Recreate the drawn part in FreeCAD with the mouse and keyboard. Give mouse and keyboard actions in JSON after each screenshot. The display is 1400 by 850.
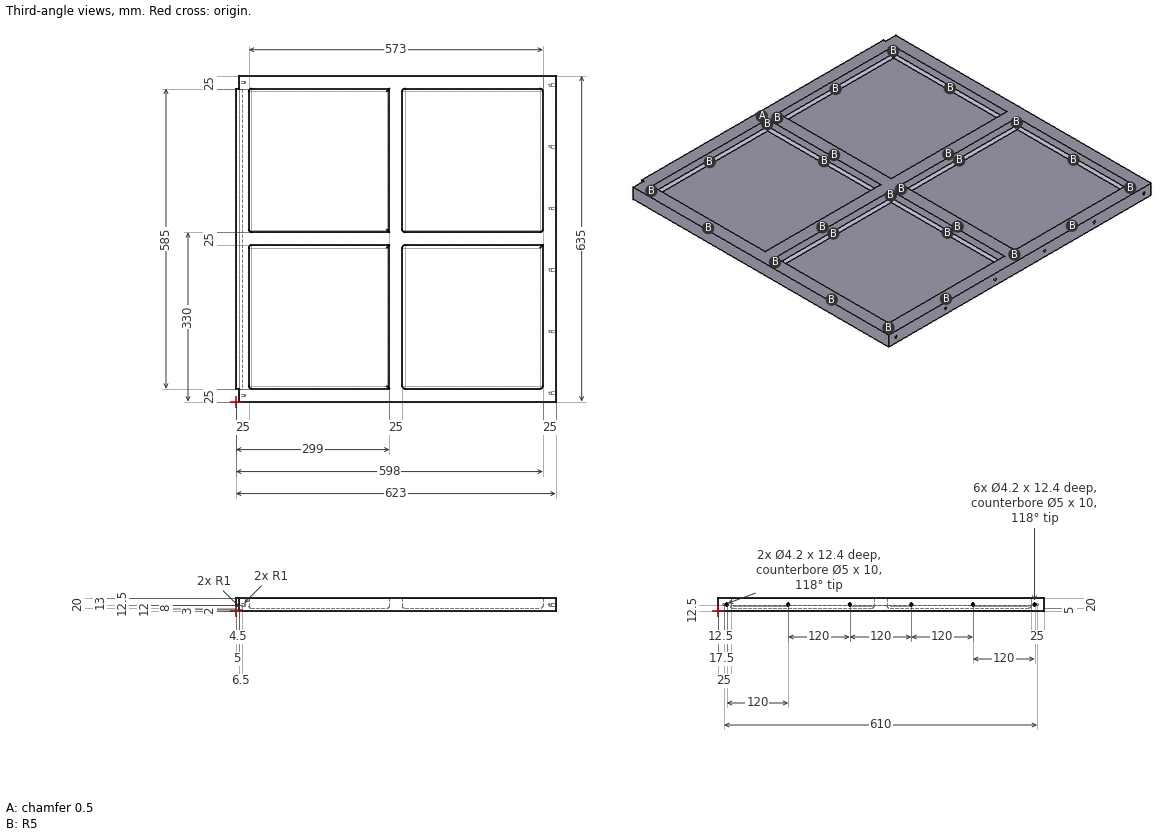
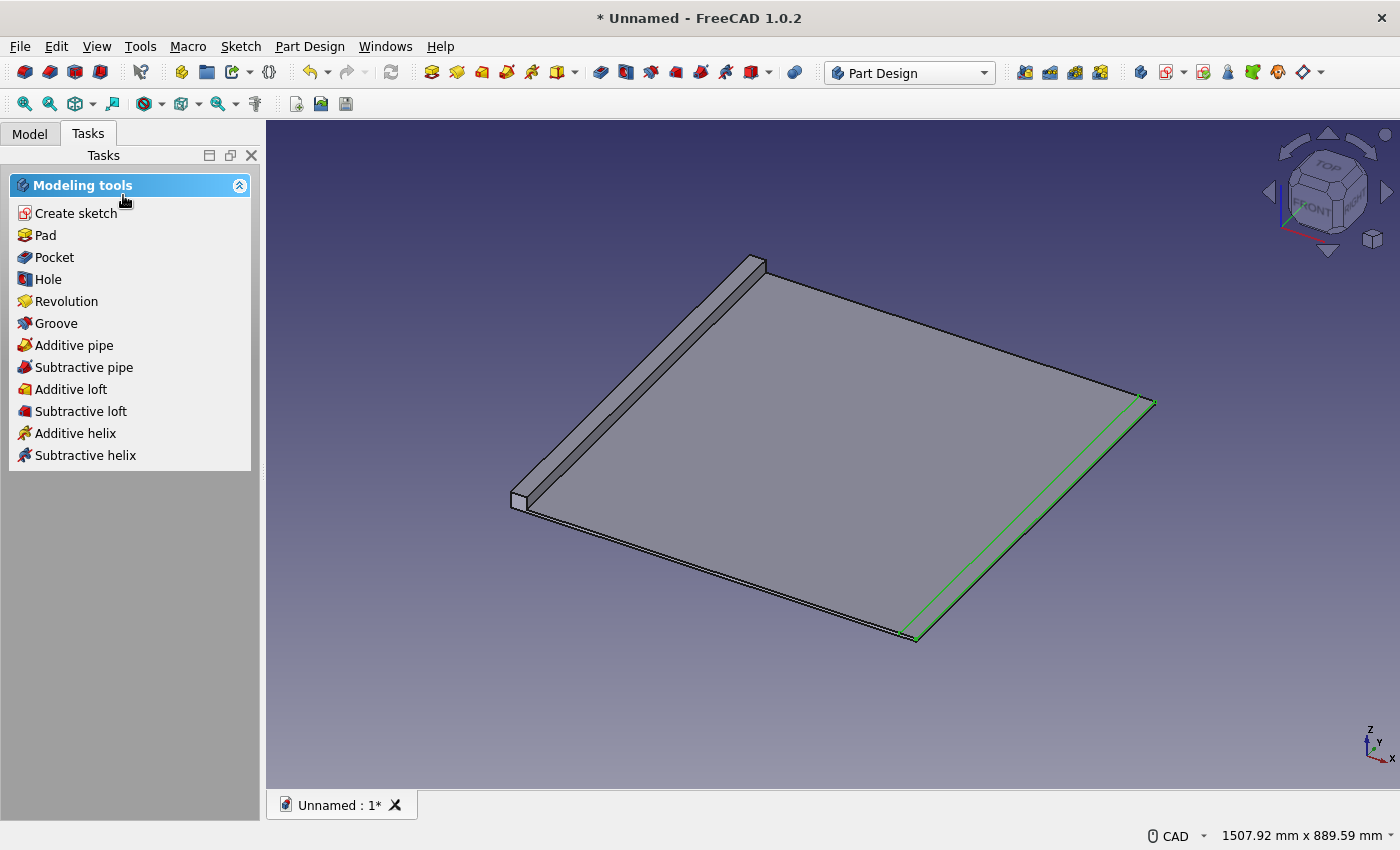
{"action": "left_click", "coordinate": [432, 72]}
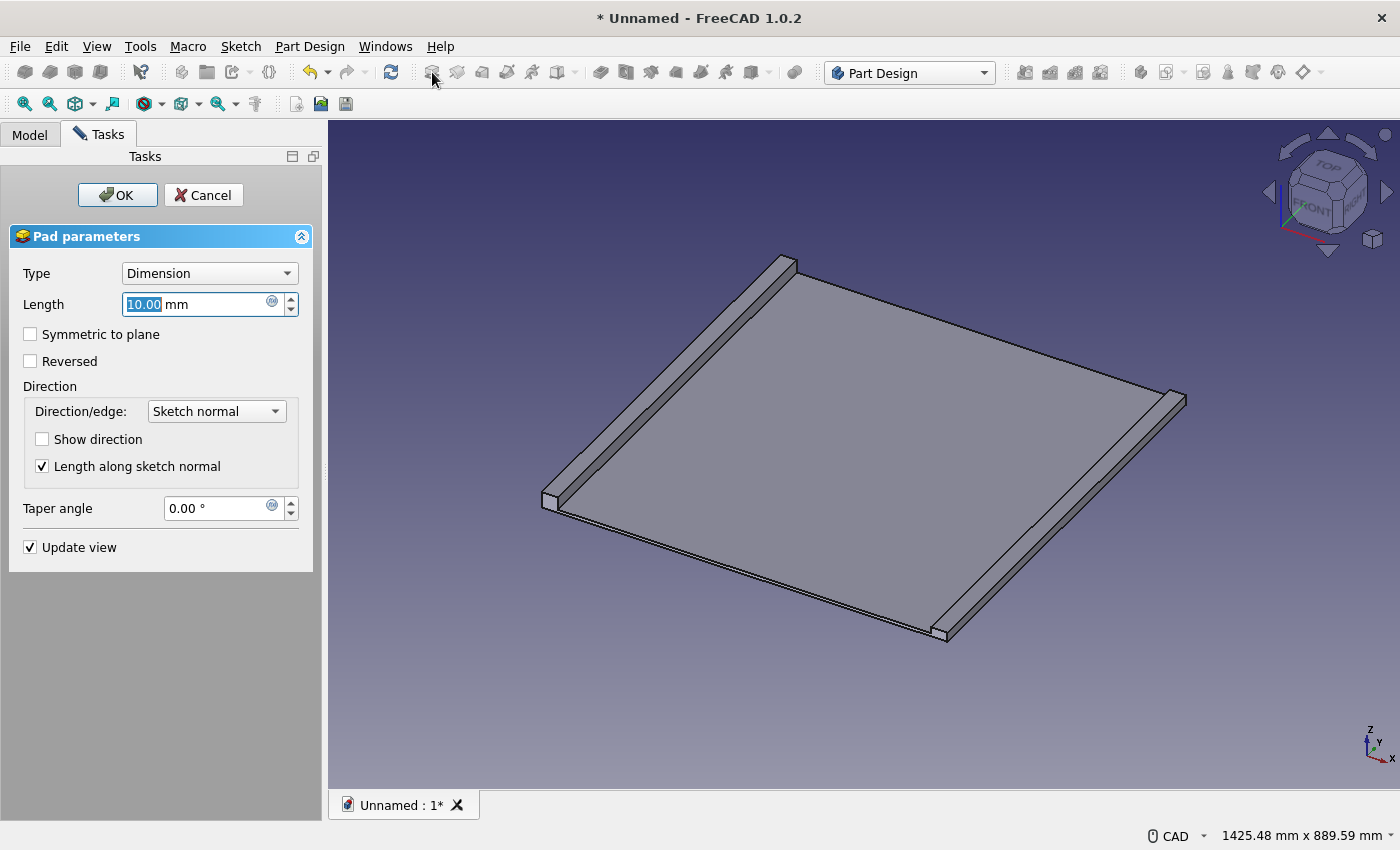
{"action": "type", "text": "20"}
{"action": "key", "text": "Tab"}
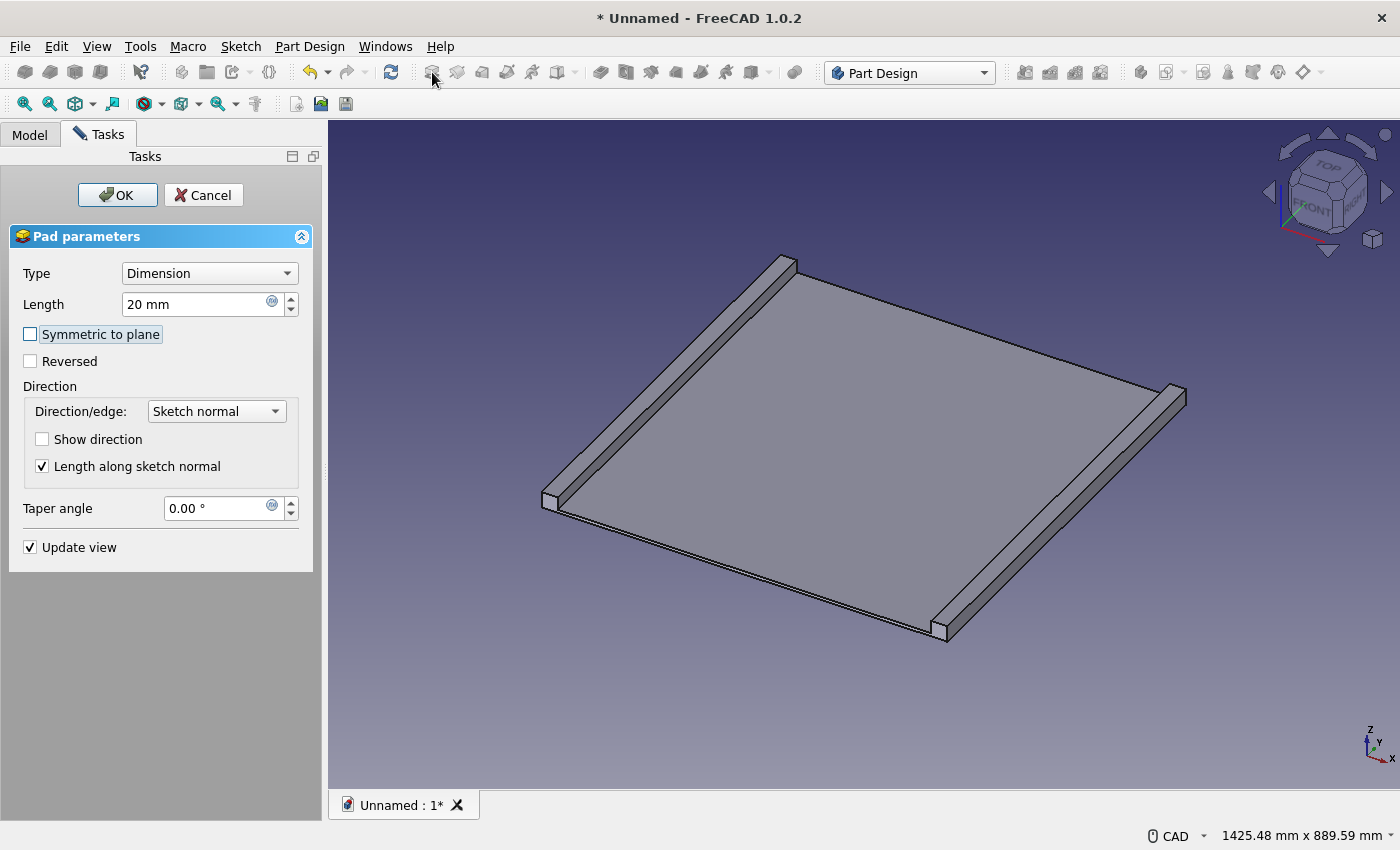
{"action": "left_click", "coordinate": [118, 195]}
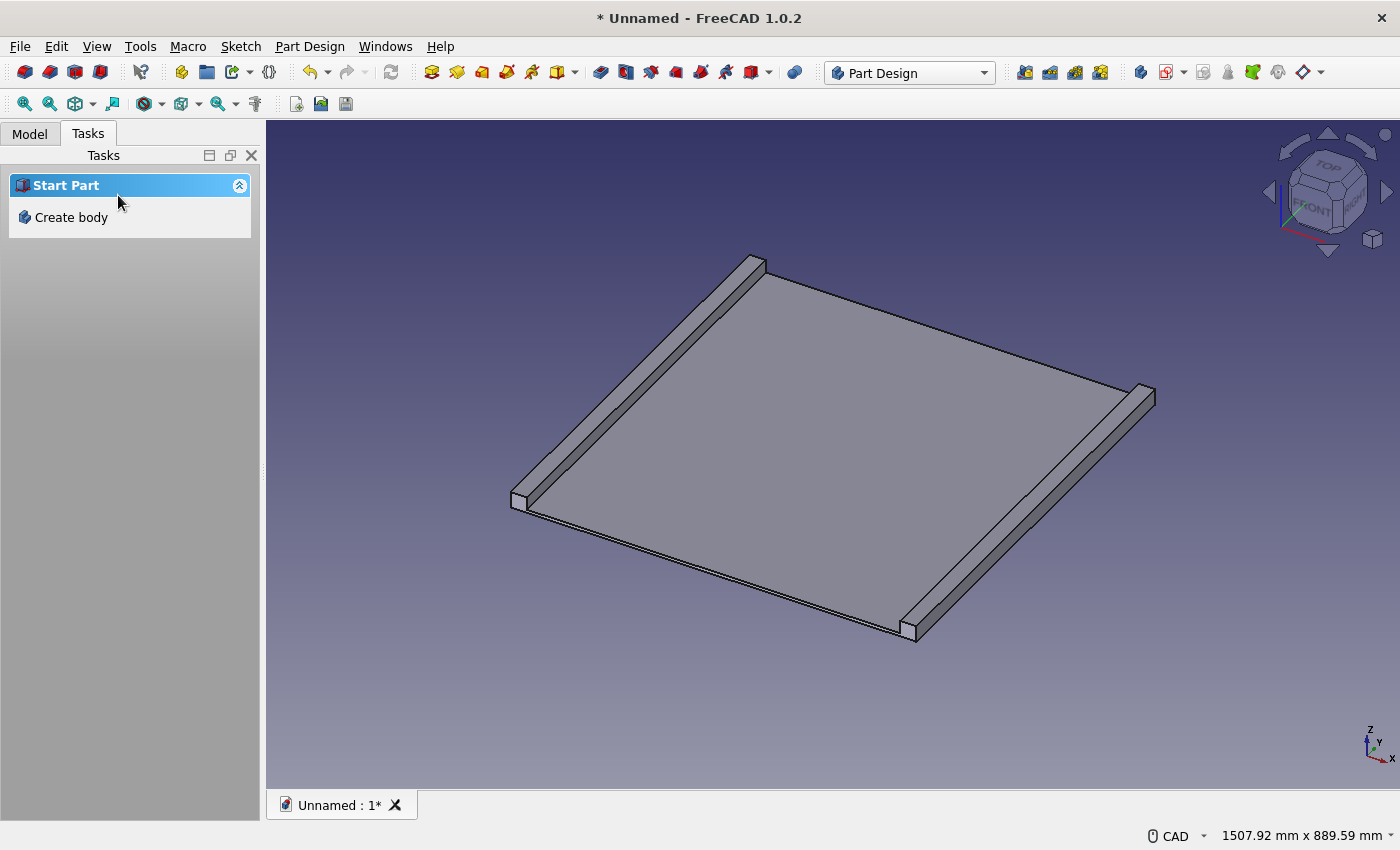
{"action": "key", "text": "4"}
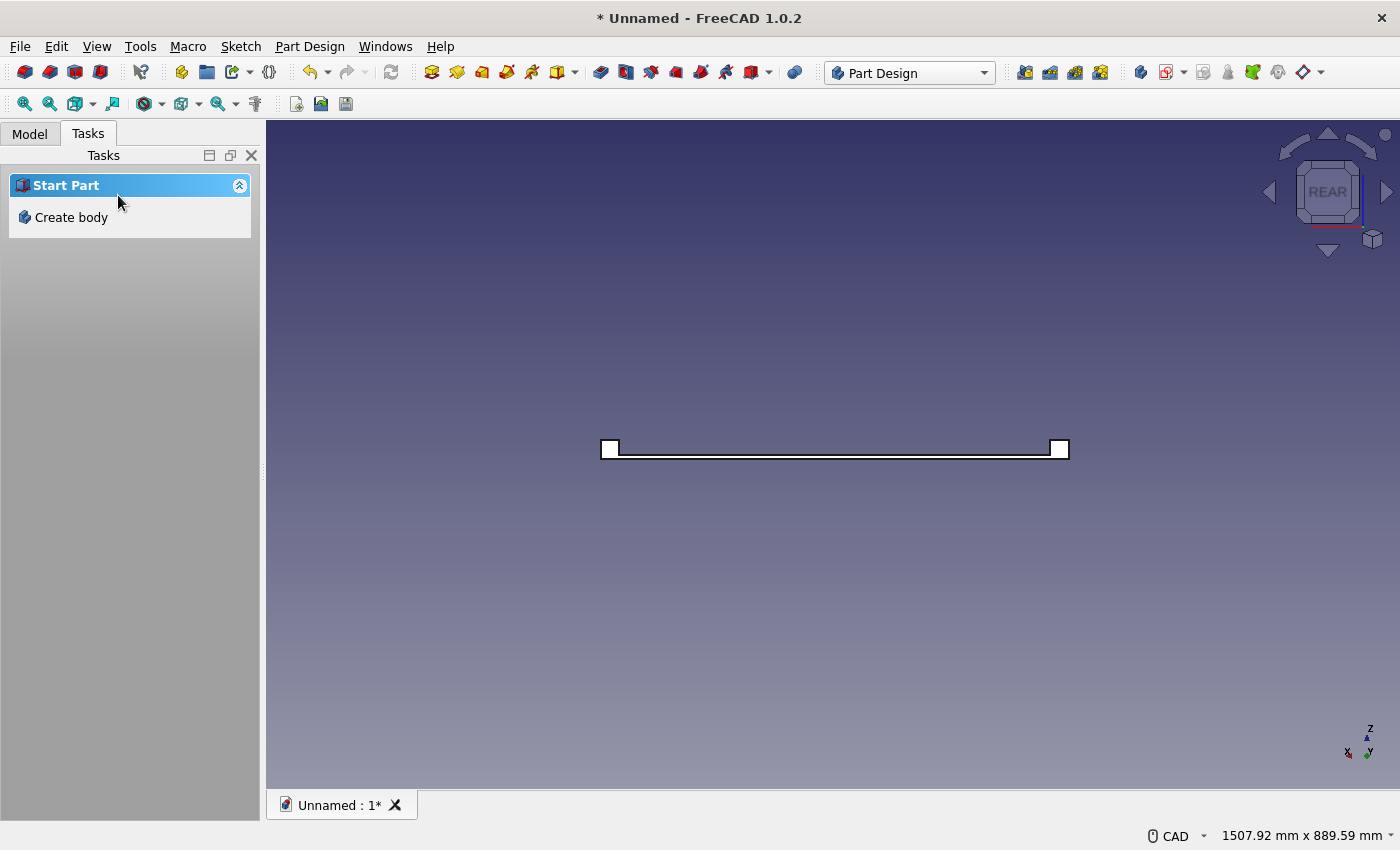
{"action": "key", "text": "v f"}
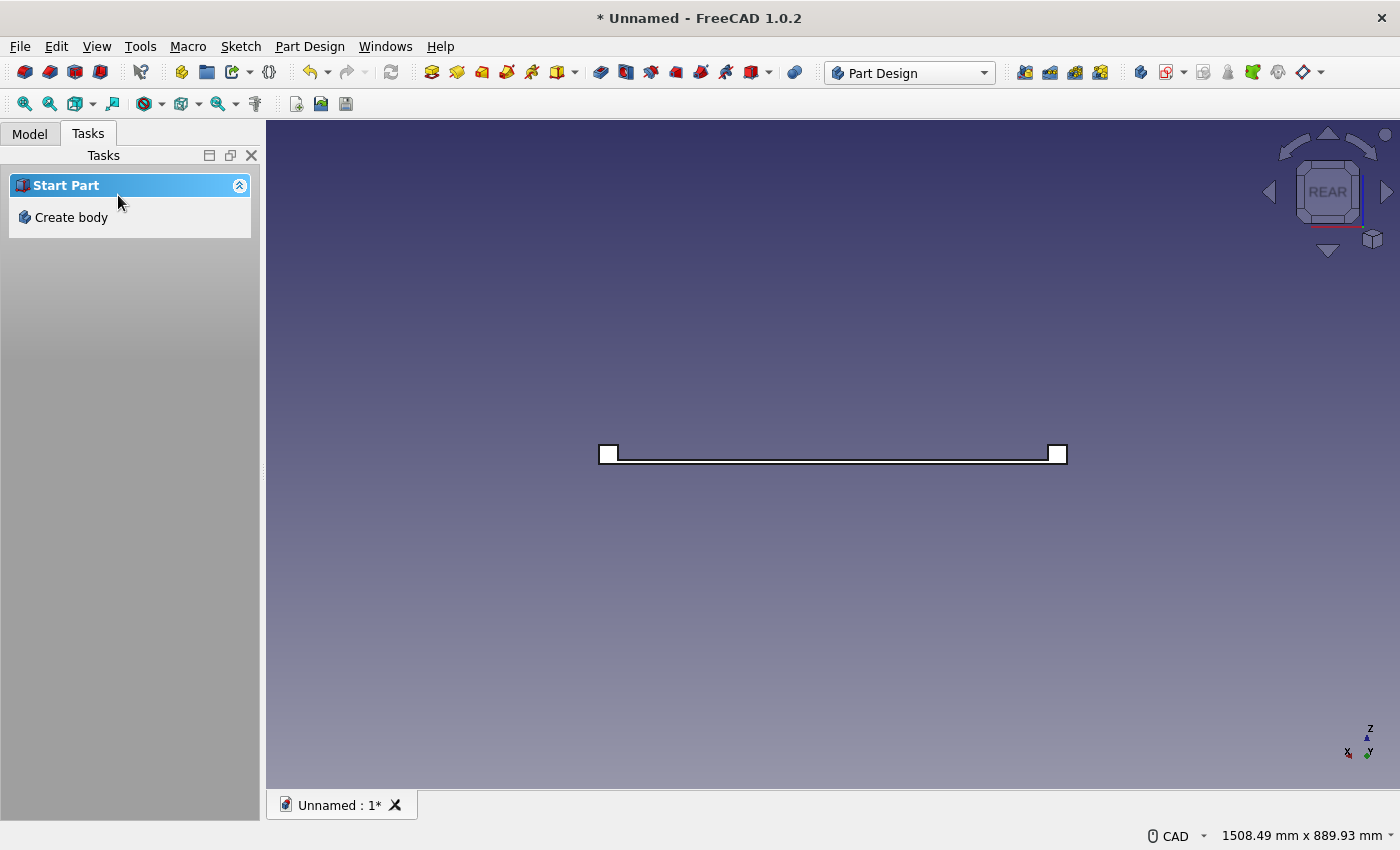
{"action": "scroll", "coordinate": [632, 462], "scroll_direction": "up", "scroll_amount": 11}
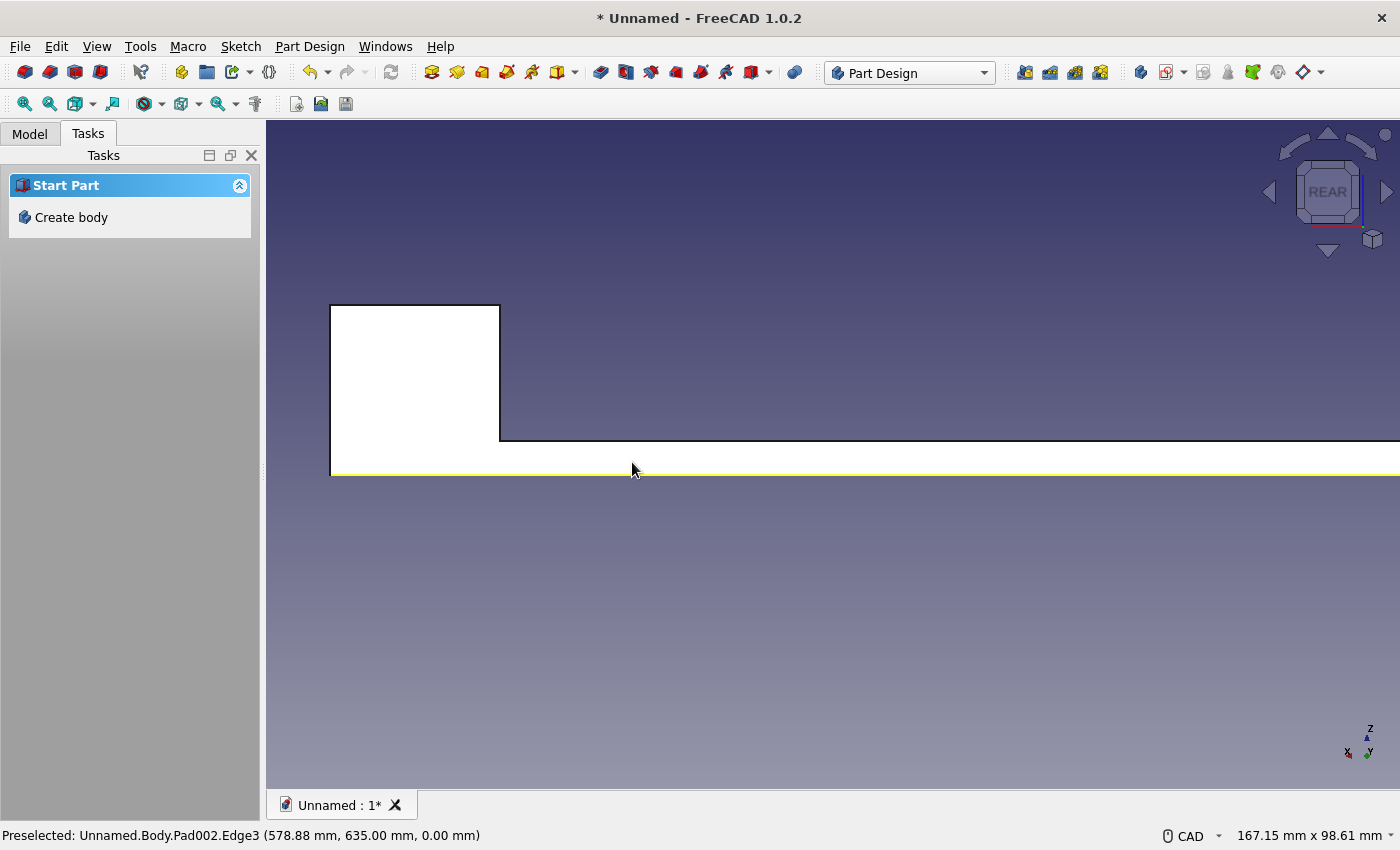
{"action": "left_click", "coordinate": [632, 462]}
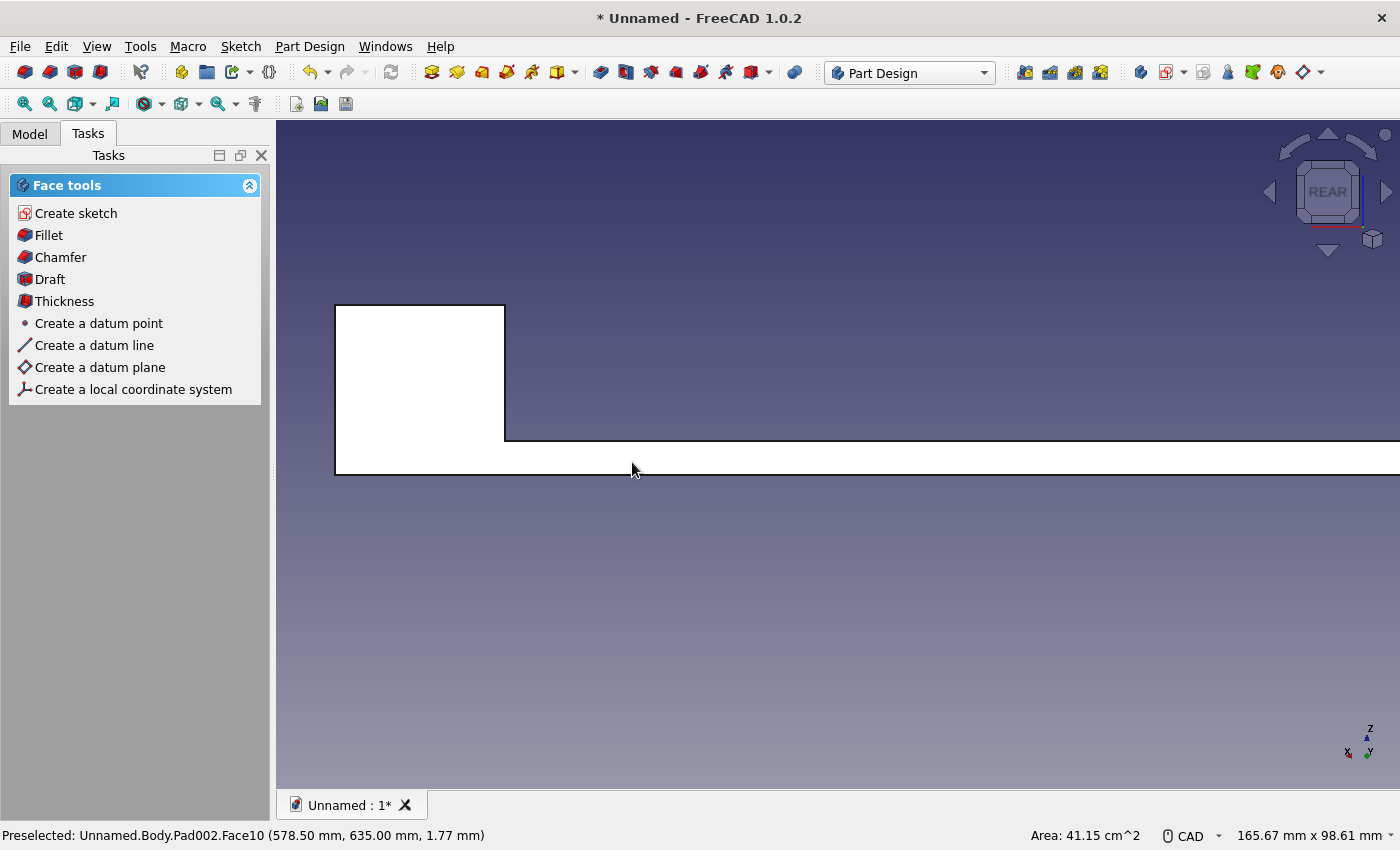
{"action": "left_click", "coordinate": [1166, 72]}